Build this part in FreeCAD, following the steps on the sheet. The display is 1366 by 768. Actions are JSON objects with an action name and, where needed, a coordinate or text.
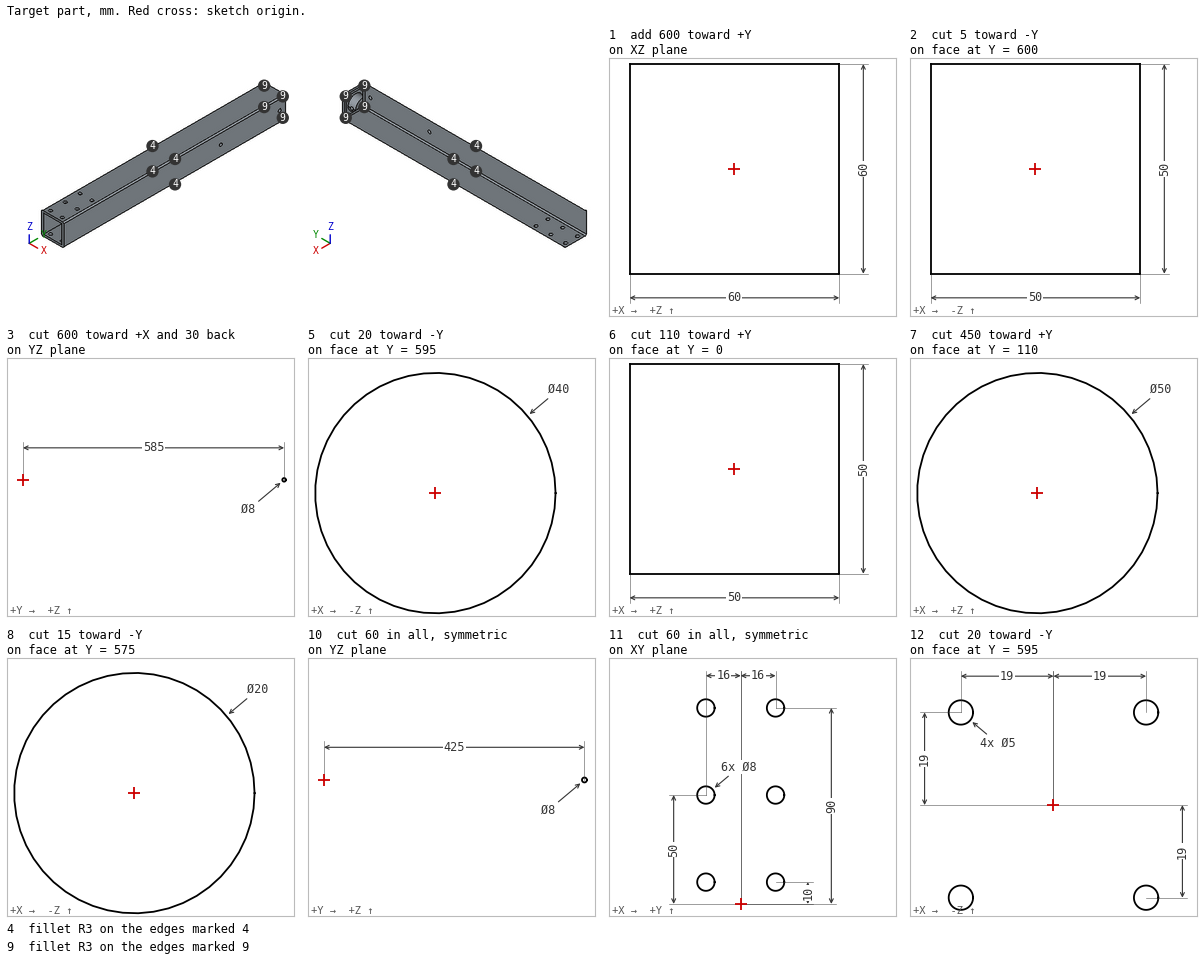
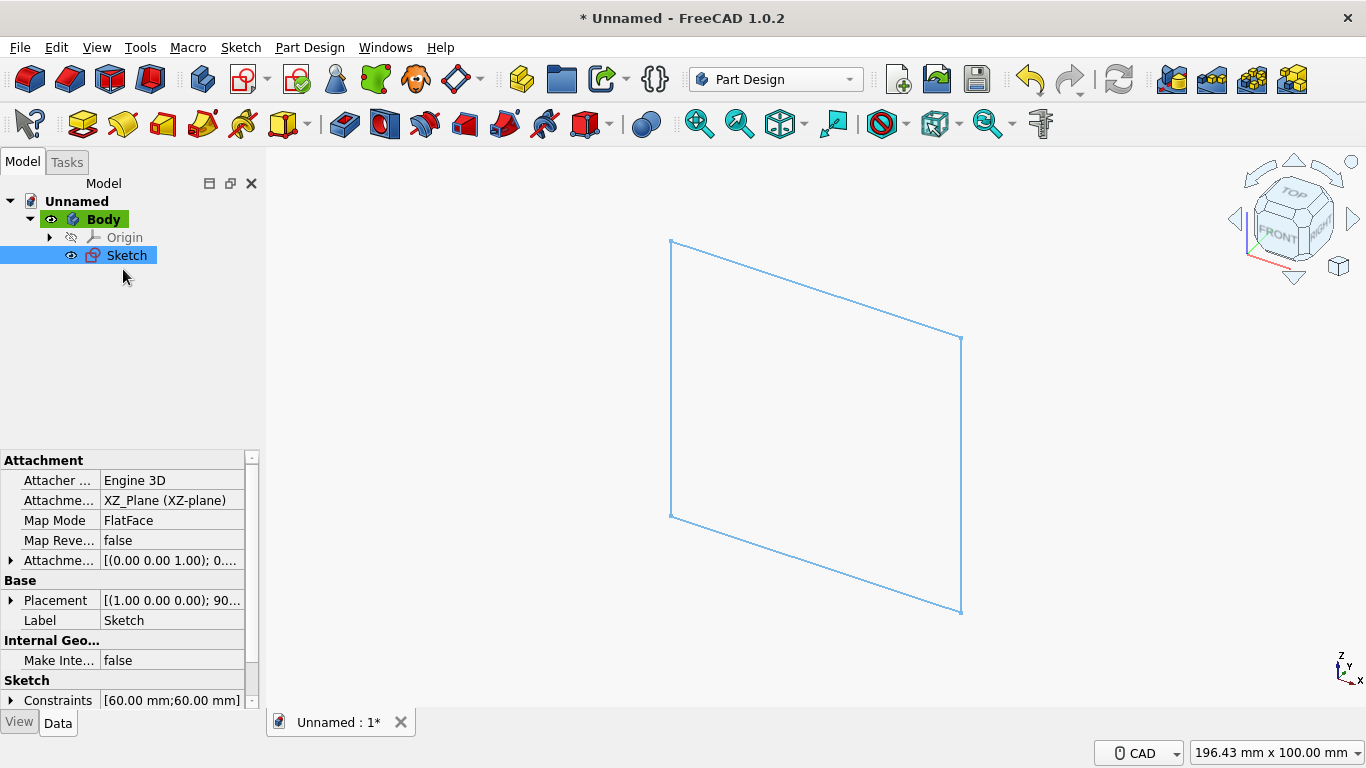
{"action": "left_click", "coordinate": [84, 124]}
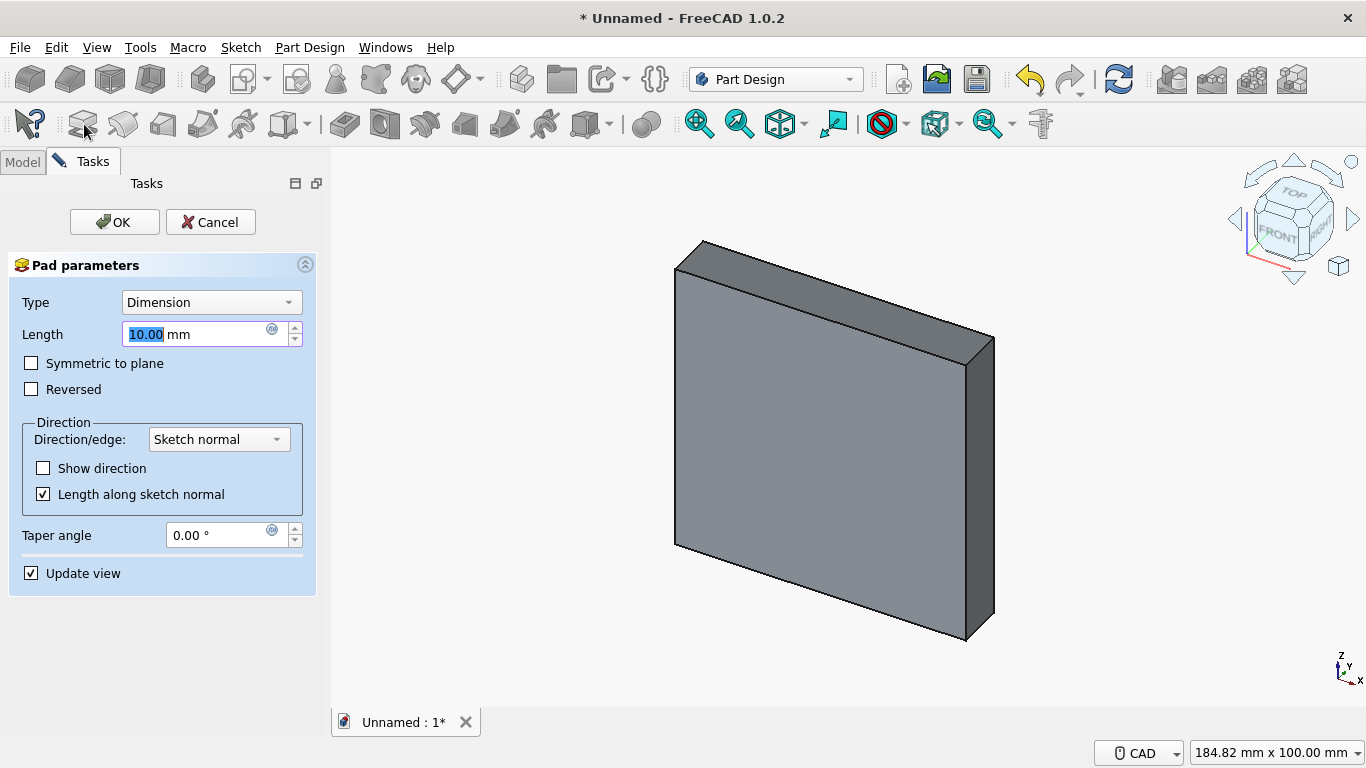
{"action": "type", "text": "600"}
{"action": "key", "text": "Tab"}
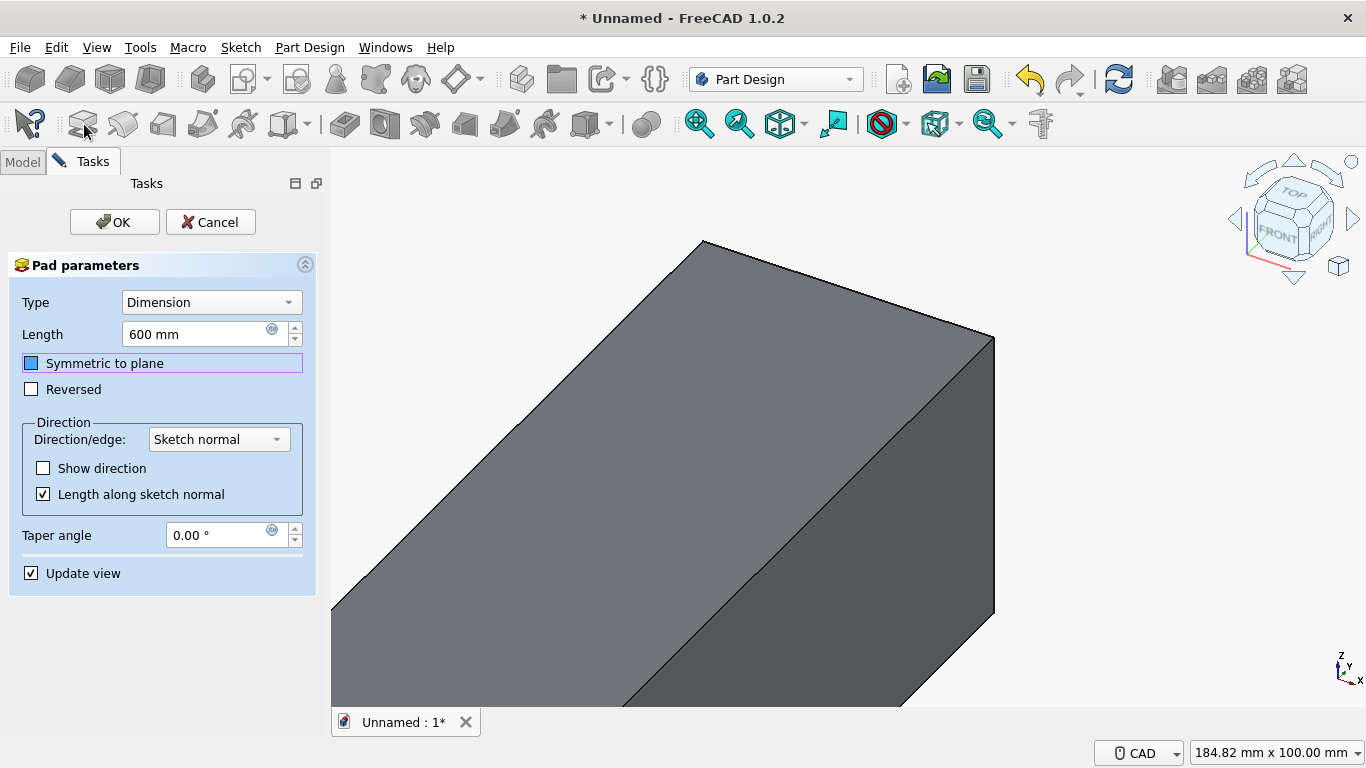
{"action": "left_click", "coordinate": [30, 389]}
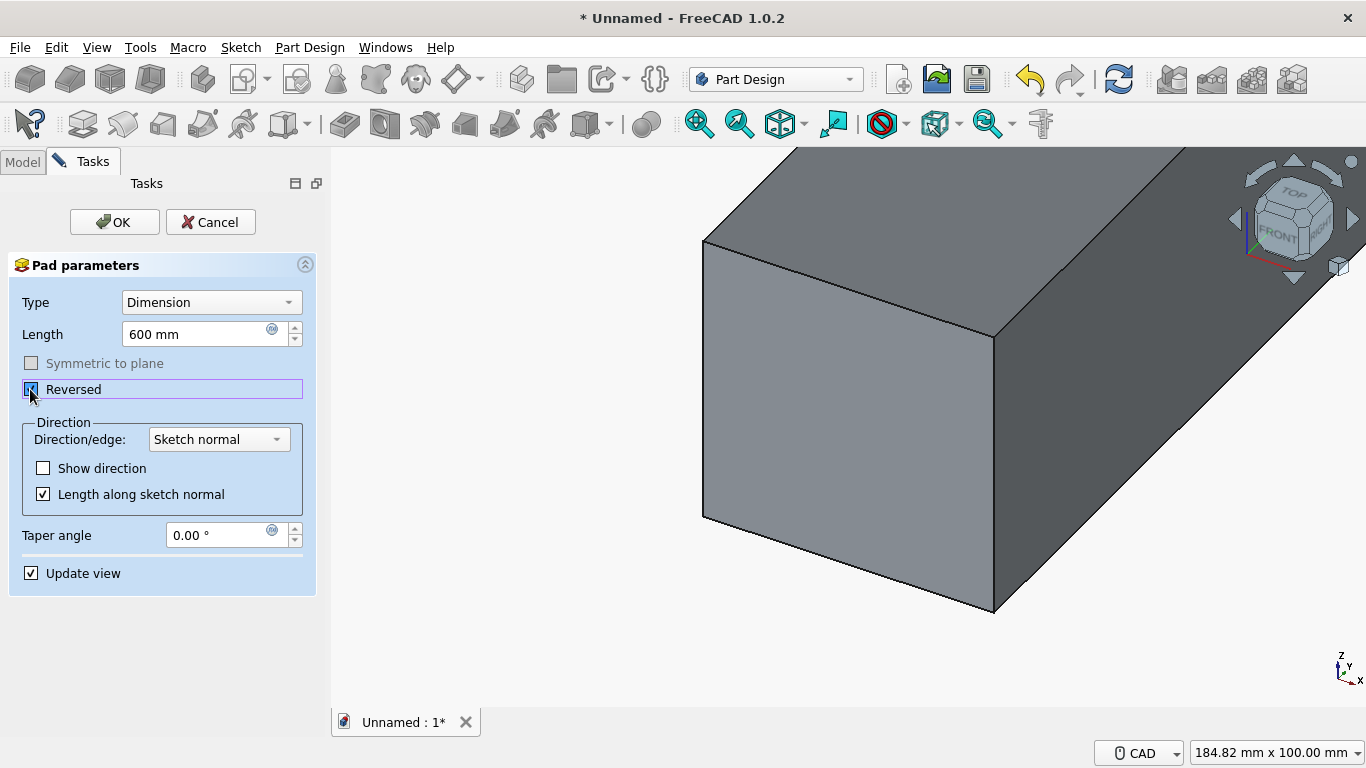
{"action": "left_click", "coordinate": [115, 222]}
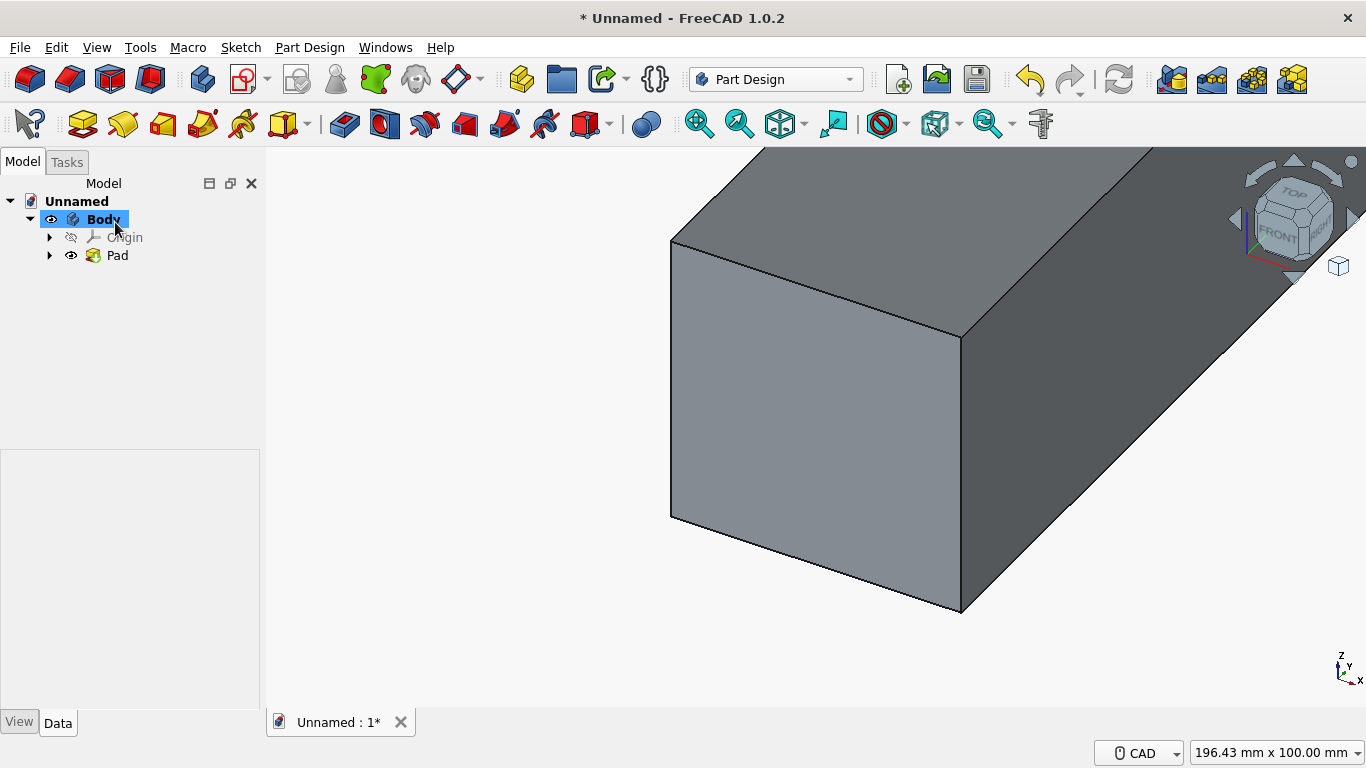
{"action": "left_click", "coordinate": [700, 124]}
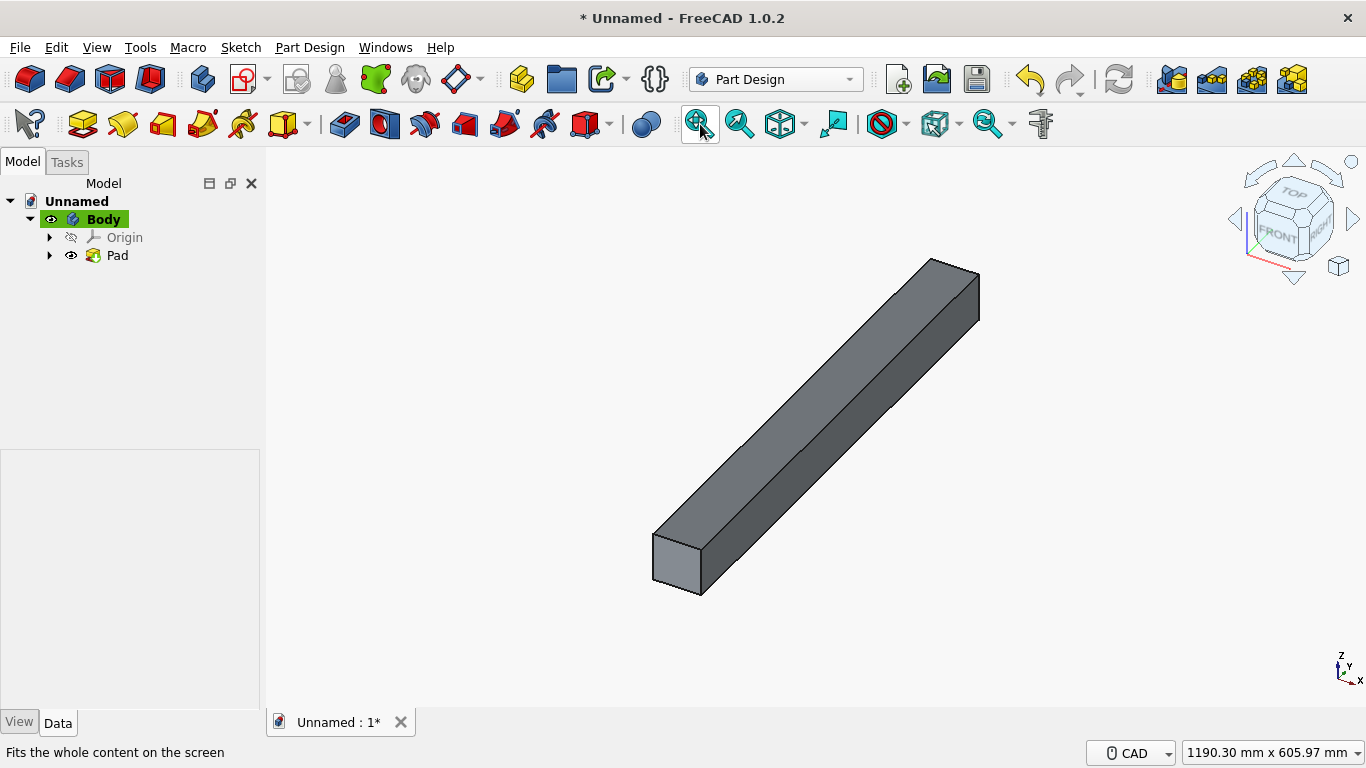
{"action": "key", "text": "4"}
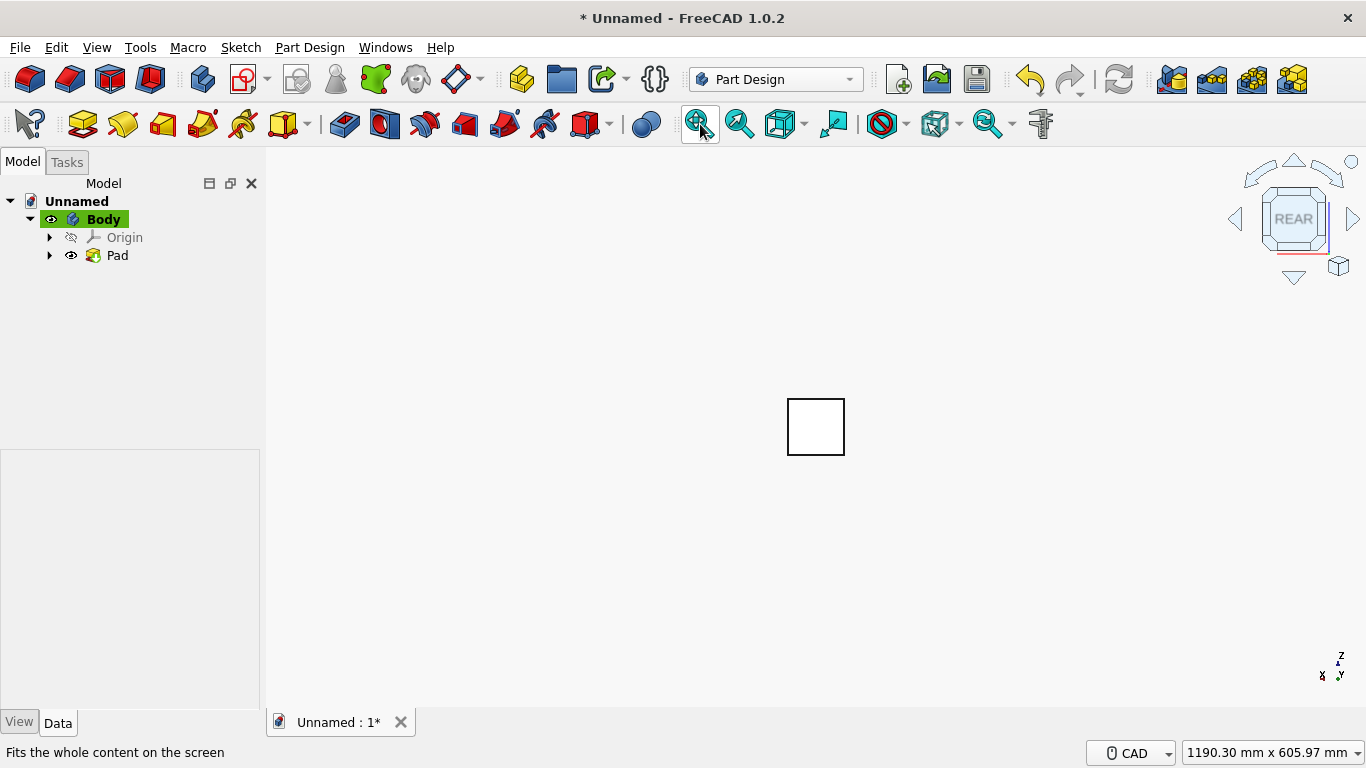
{"action": "left_click", "coordinate": [700, 124]}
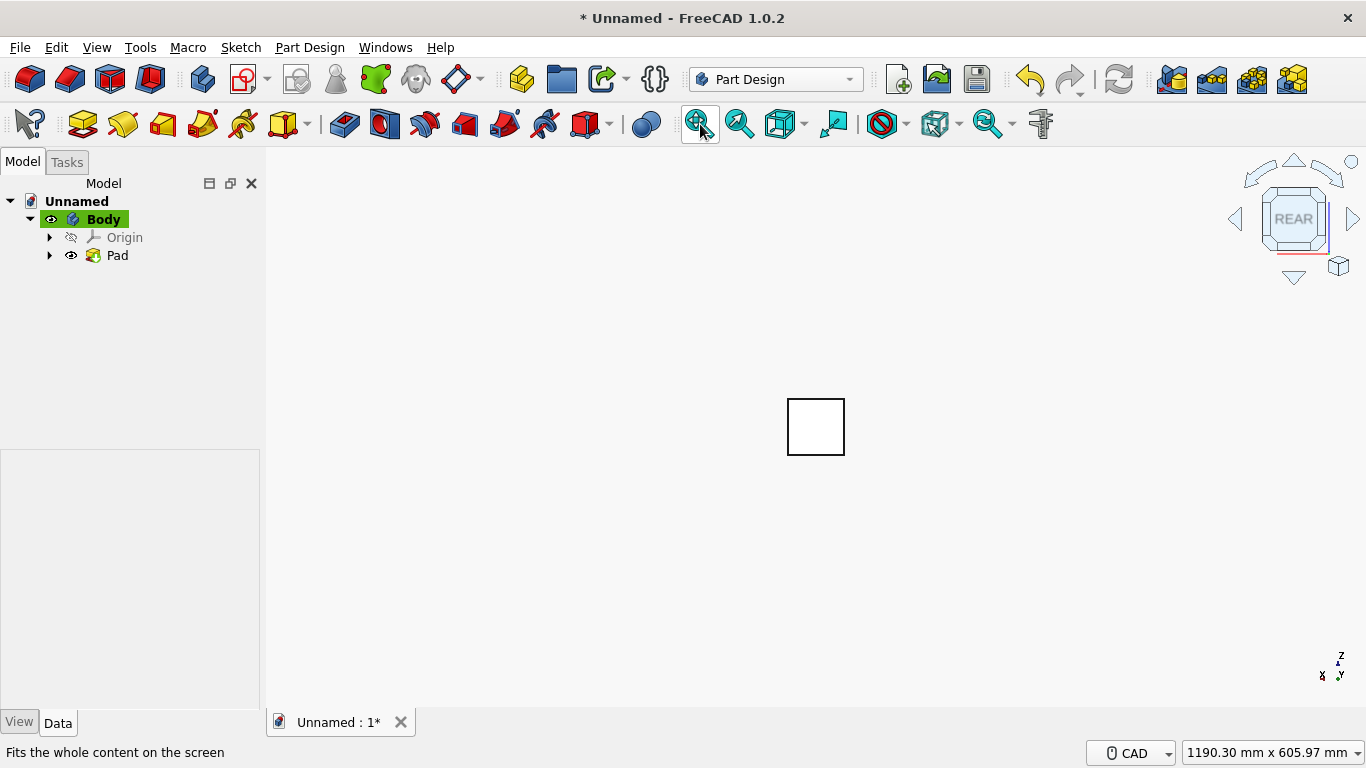
{"action": "left_click", "coordinate": [816, 426]}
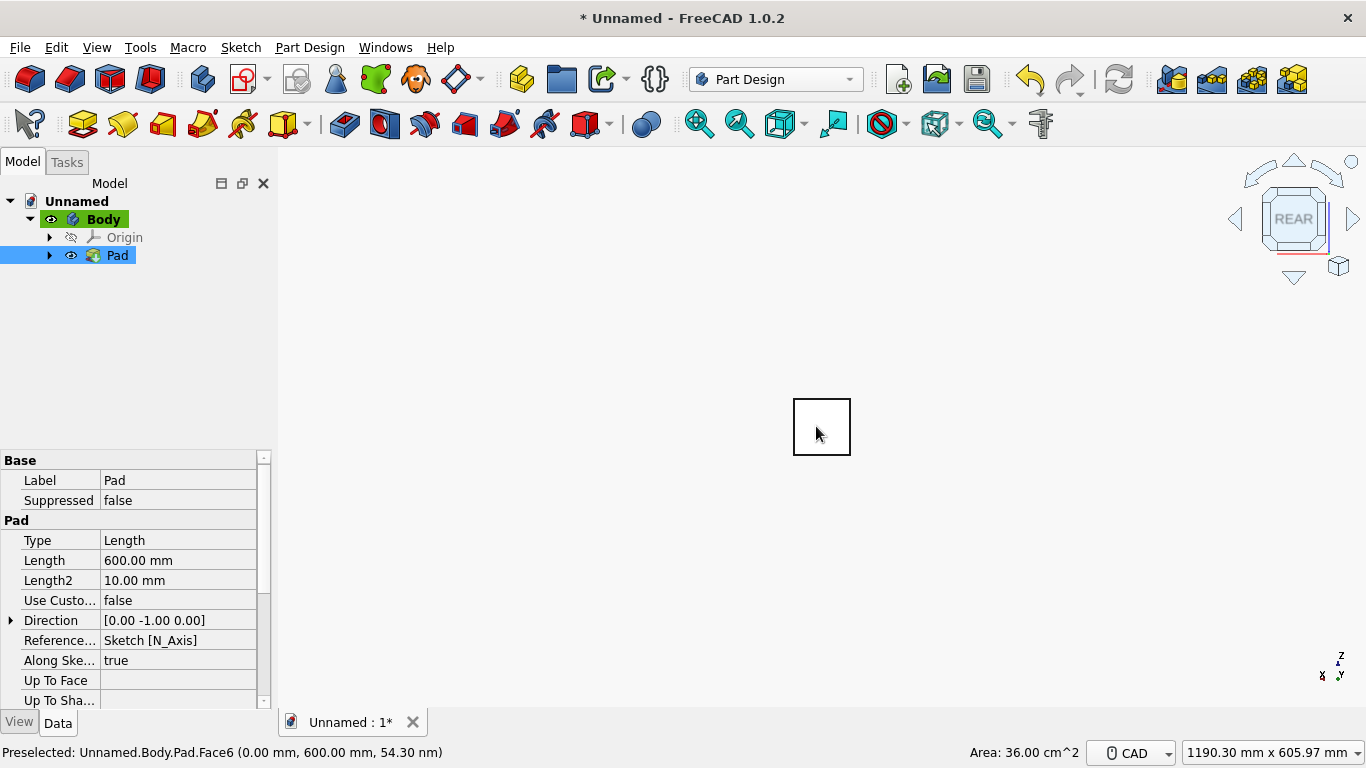
{"action": "left_click", "coordinate": [244, 80]}